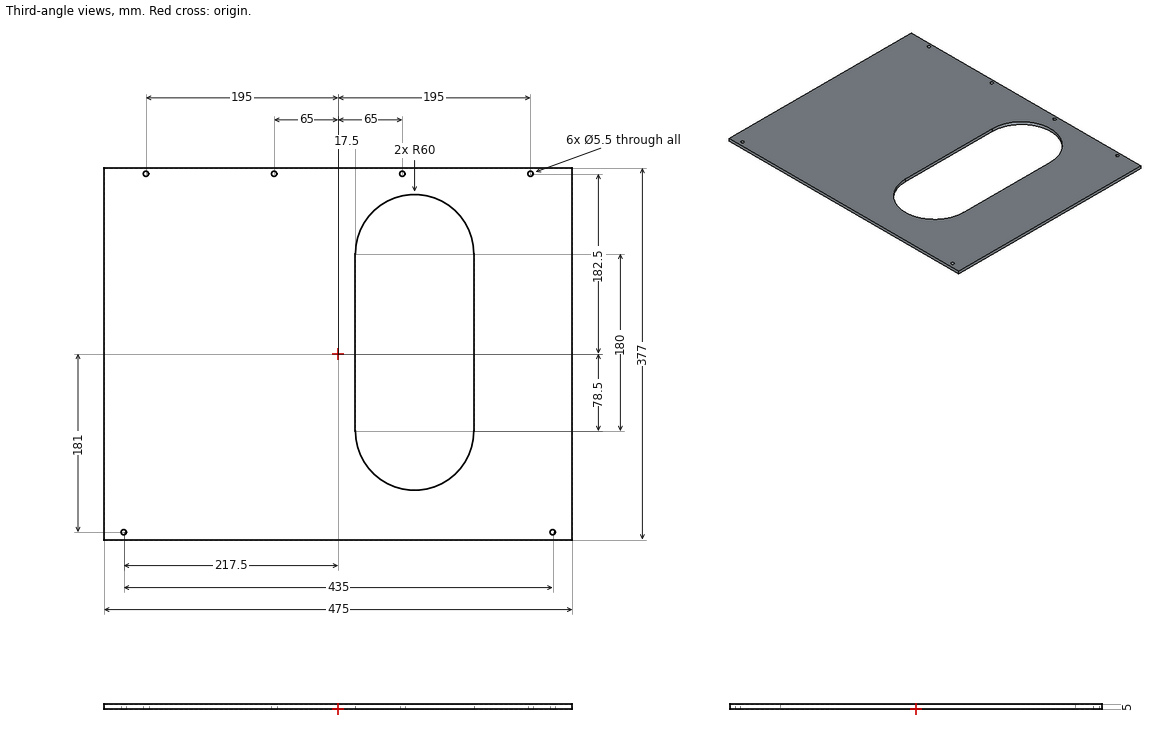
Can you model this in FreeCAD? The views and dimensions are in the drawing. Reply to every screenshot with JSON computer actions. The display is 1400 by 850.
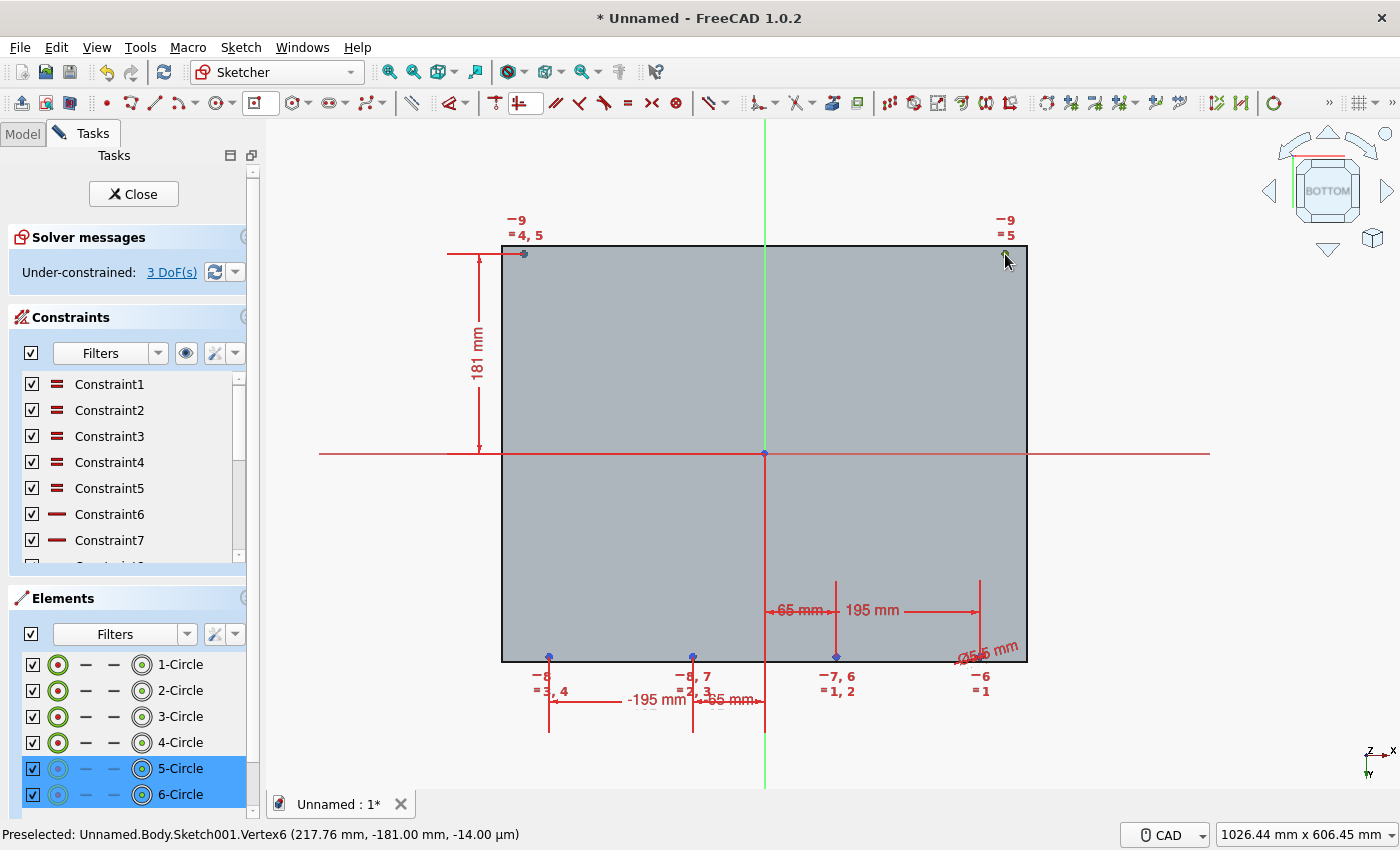
{"action": "key", "text": "l"}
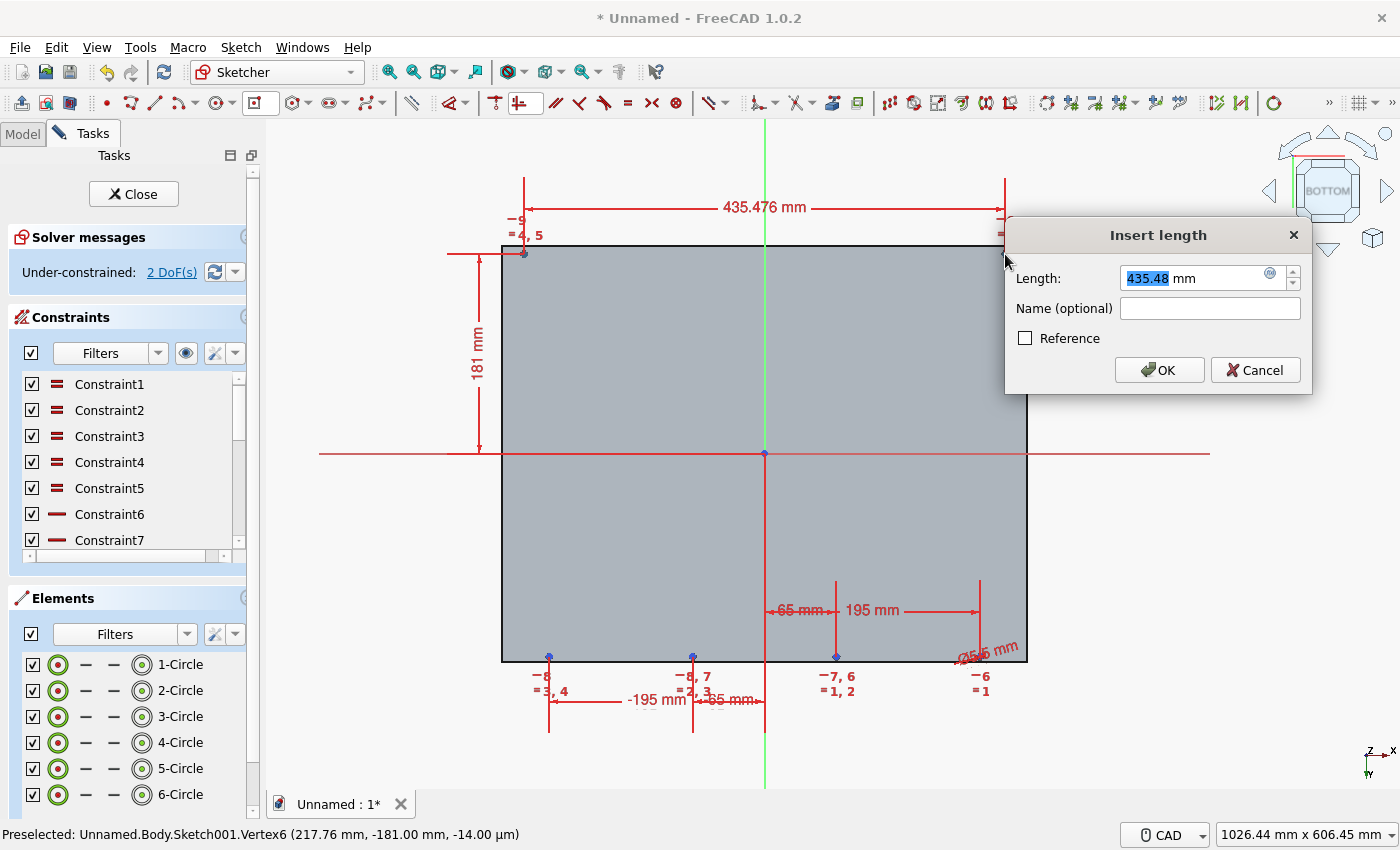
{"action": "type", "text": "435"}
{"action": "key", "text": "Return"}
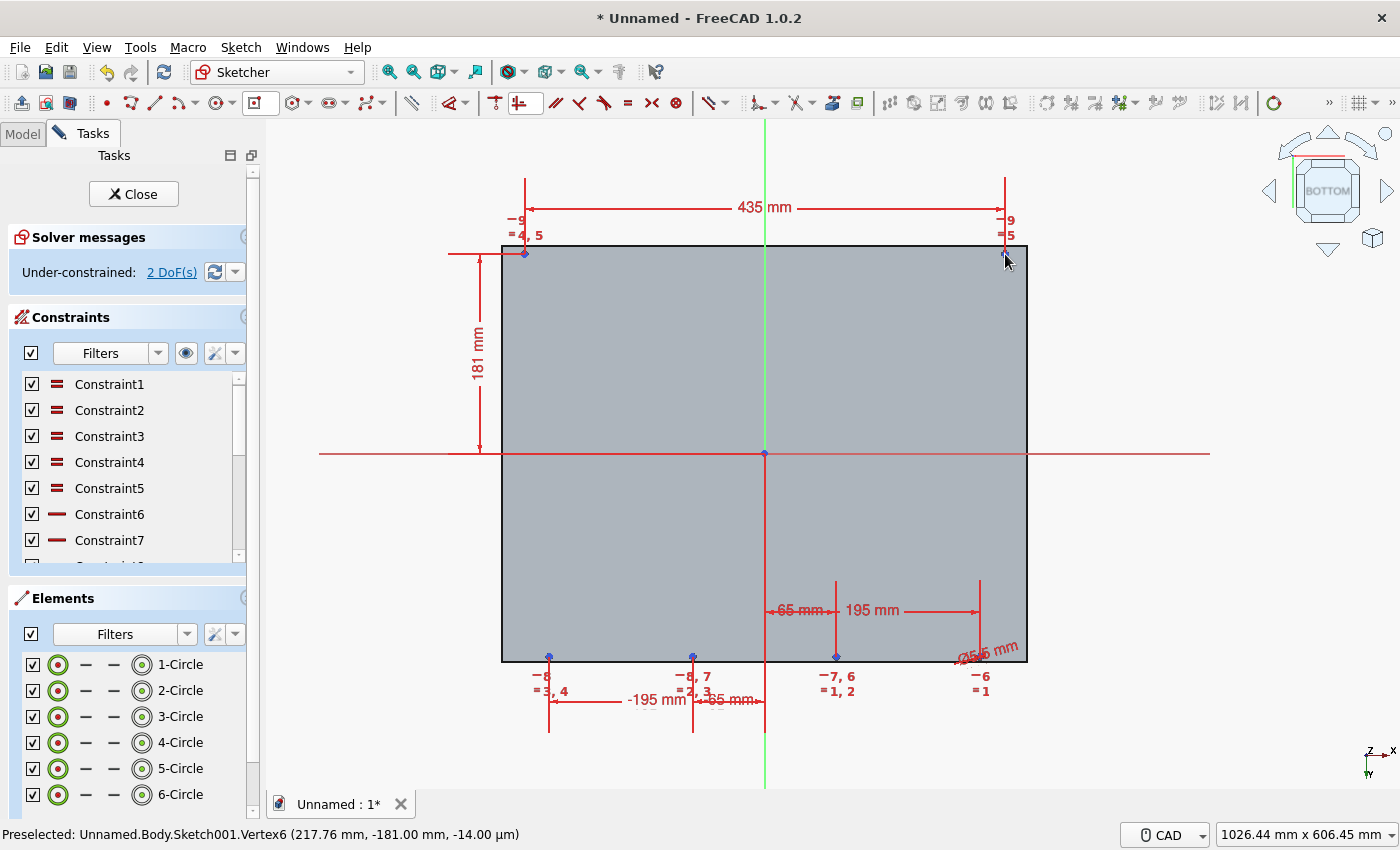
{"action": "left_click", "coordinate": [980, 657]}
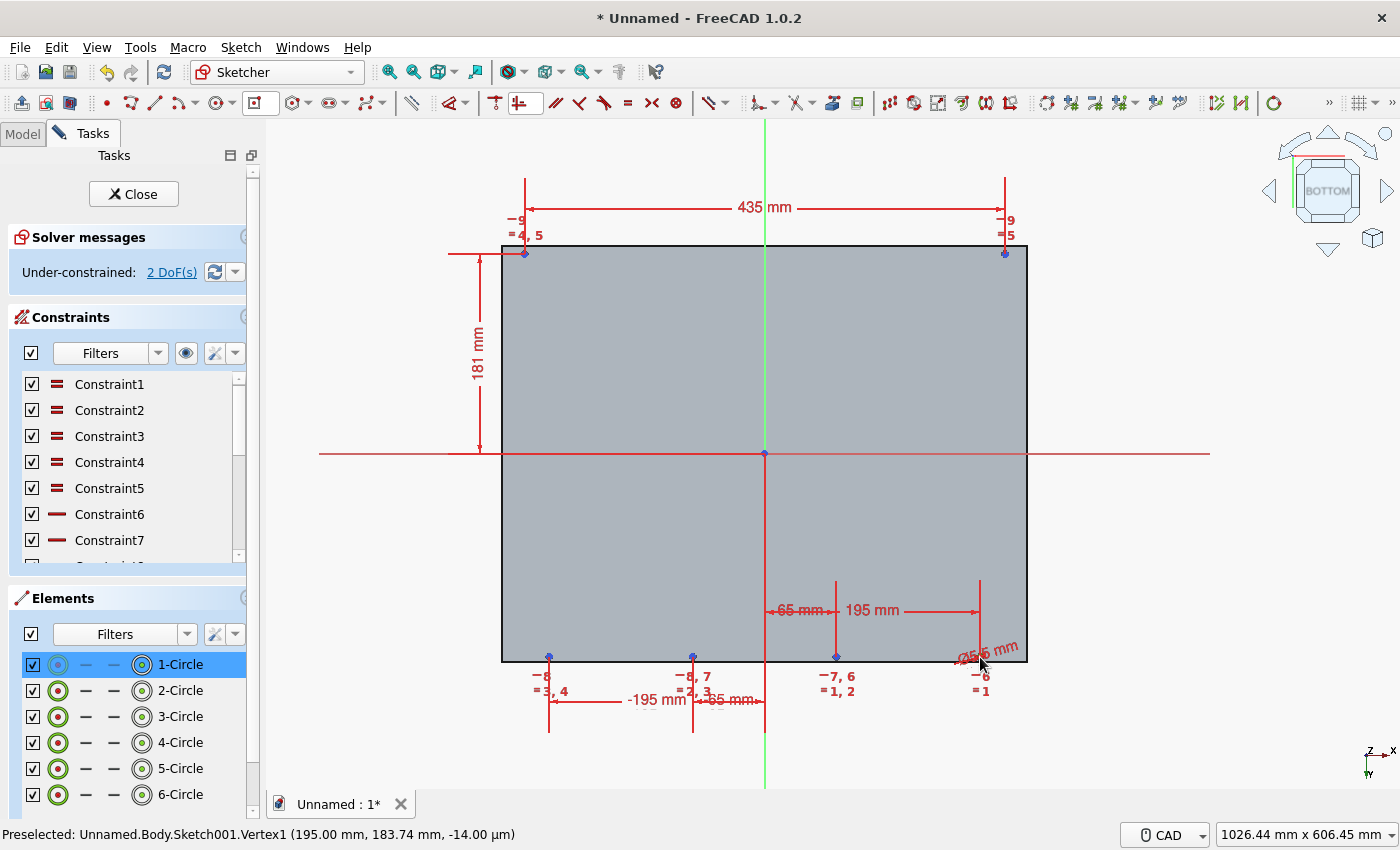
{"action": "key", "text": "i"}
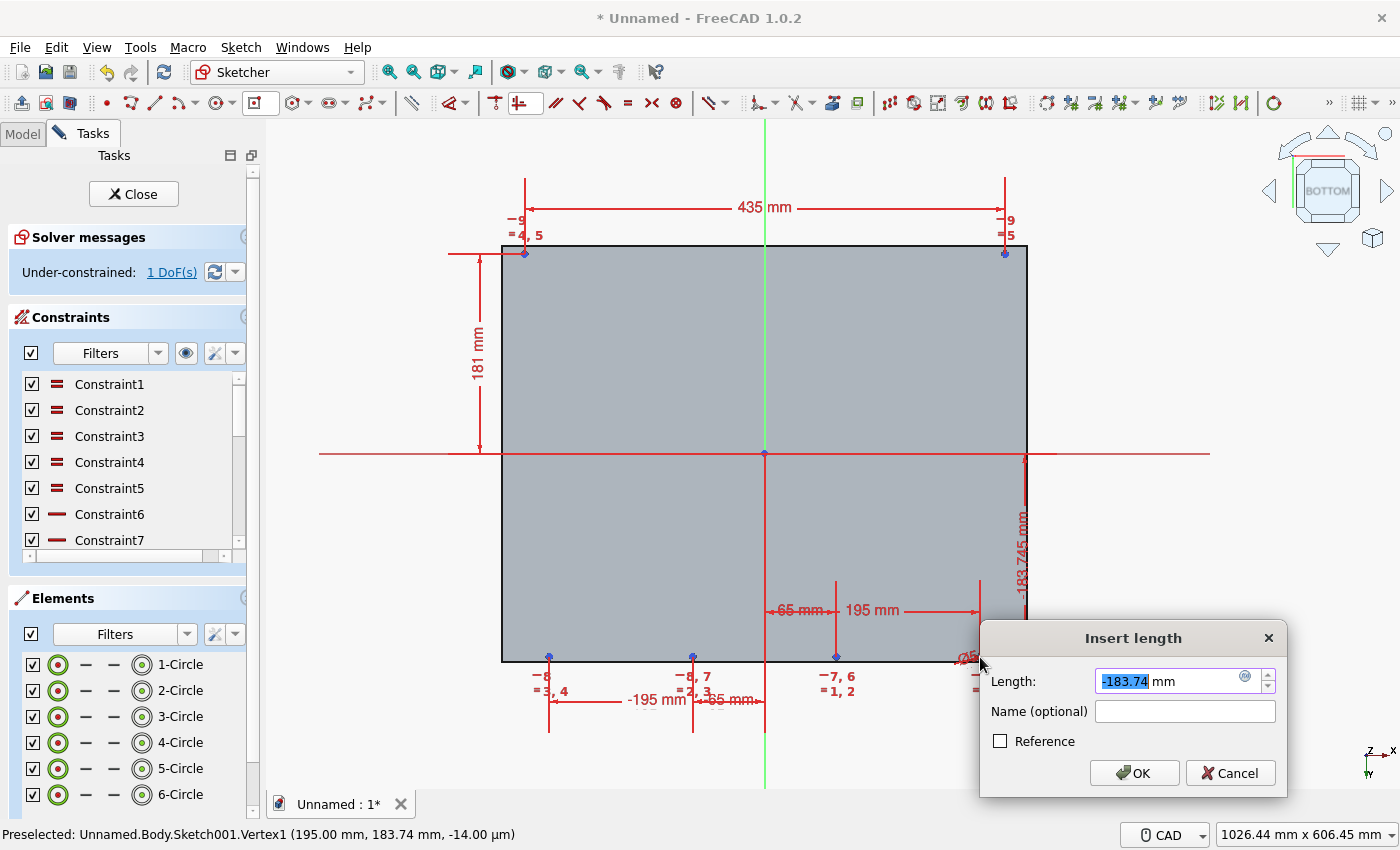
{"action": "type", "text": "-182.5"}
{"action": "key", "text": "Return"}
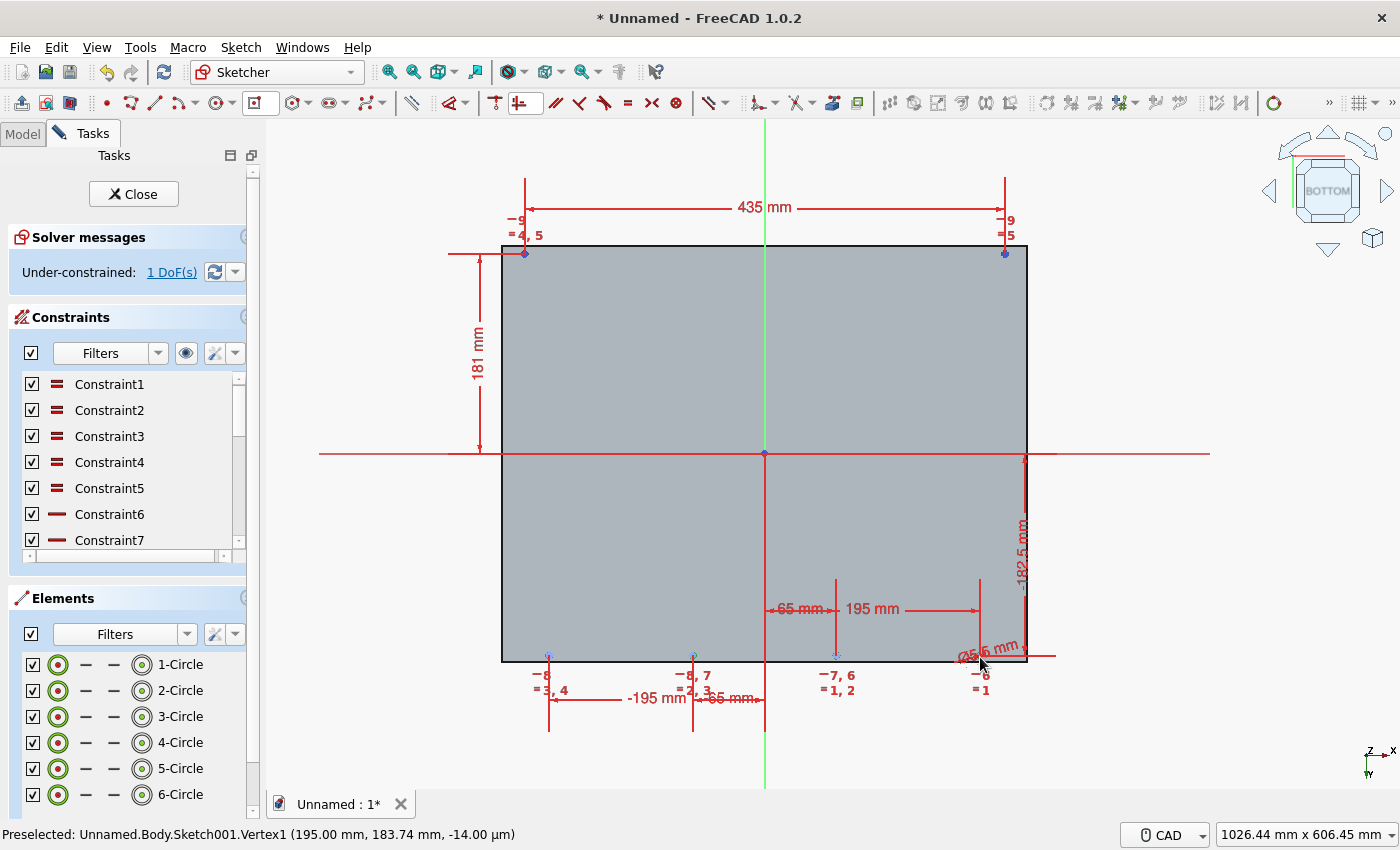
{"action": "left_click", "coordinate": [525, 254]}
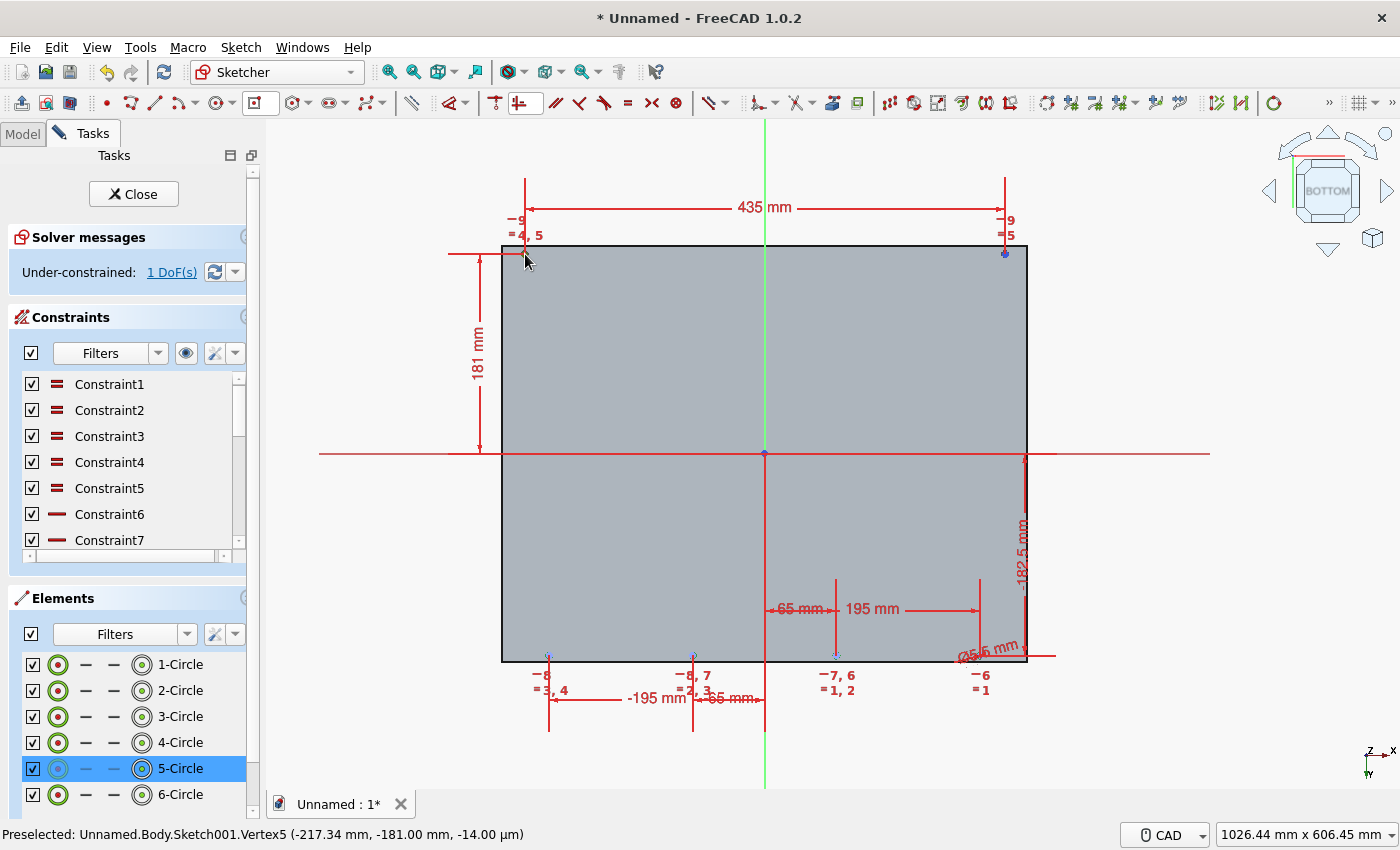
{"action": "key", "text": "l"}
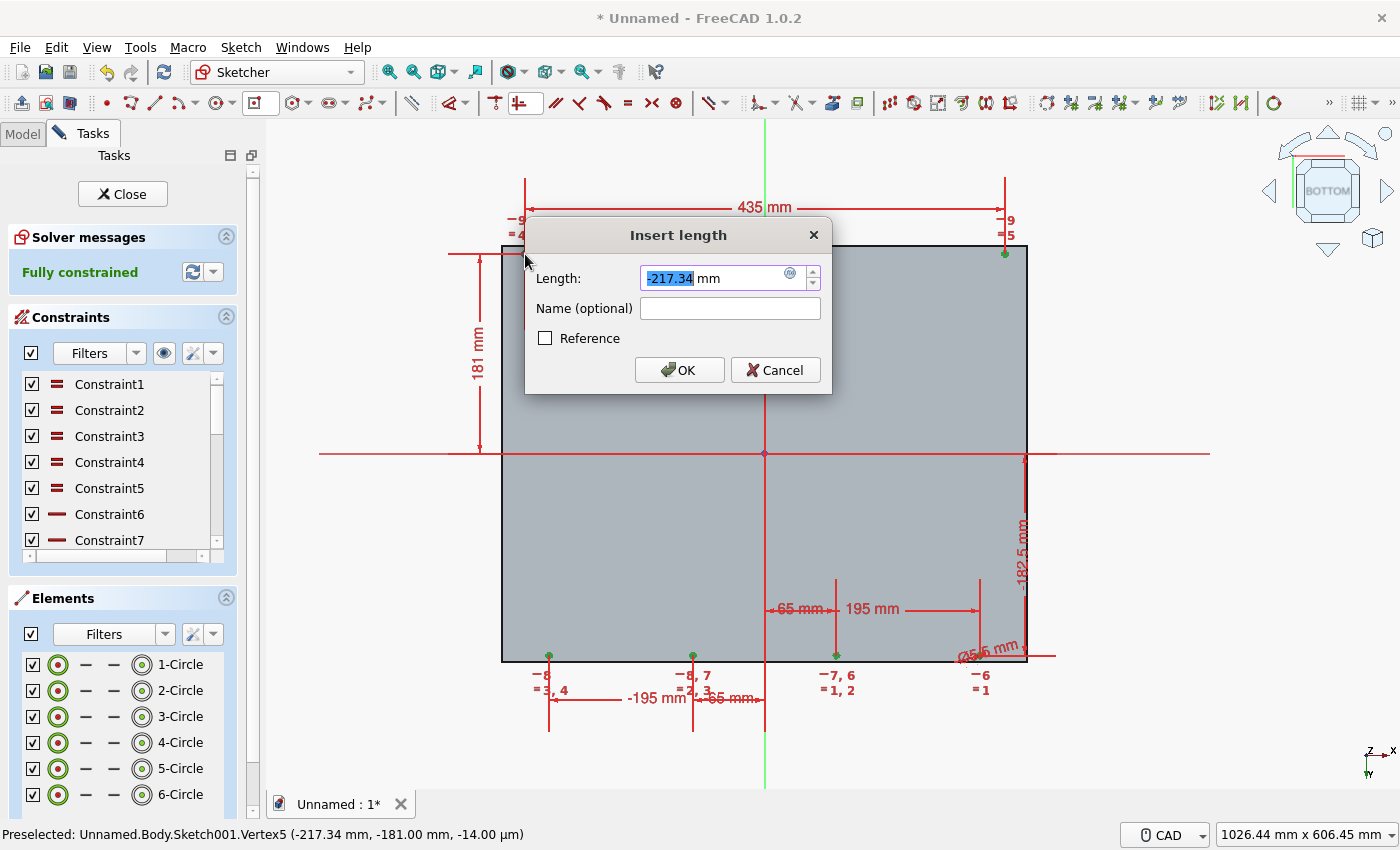
{"action": "type", "text": "-217.5"}
{"action": "key", "text": "Return"}